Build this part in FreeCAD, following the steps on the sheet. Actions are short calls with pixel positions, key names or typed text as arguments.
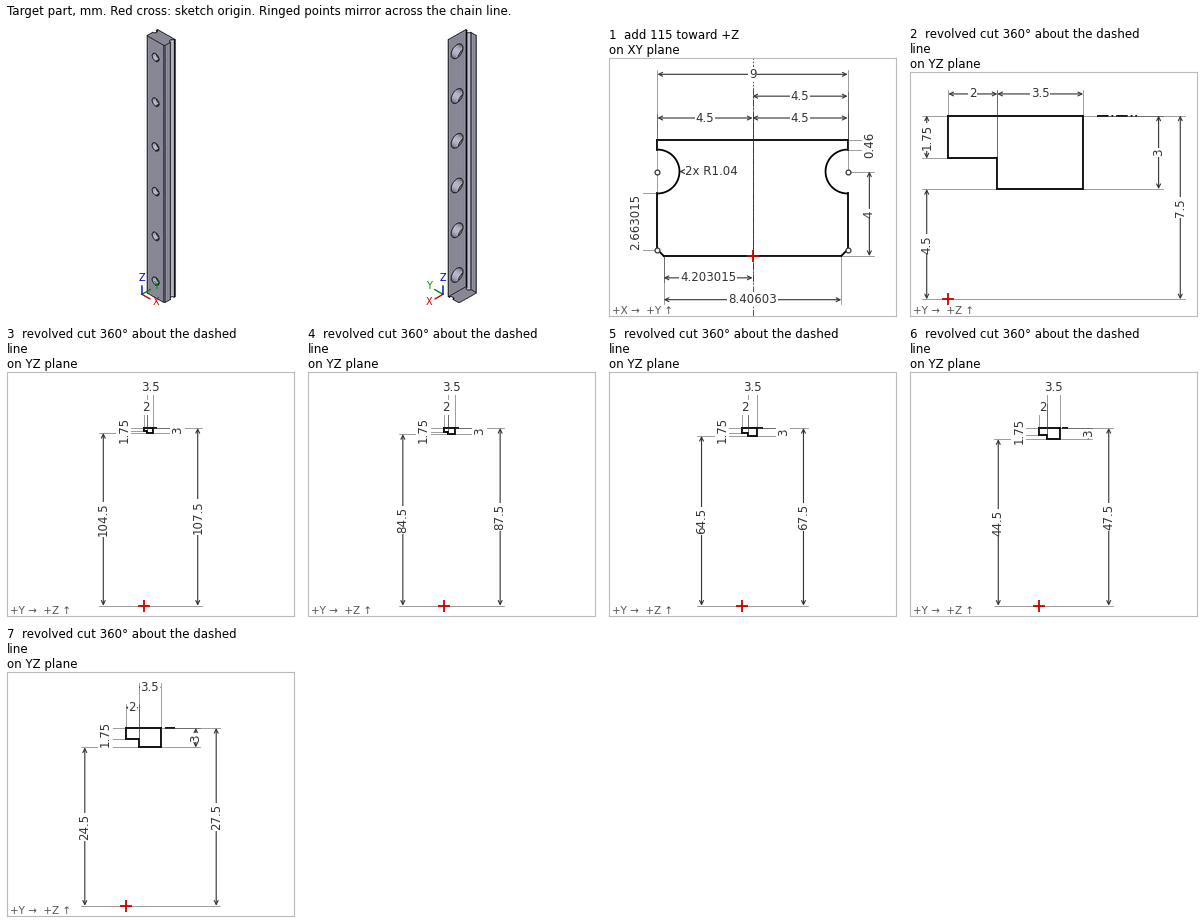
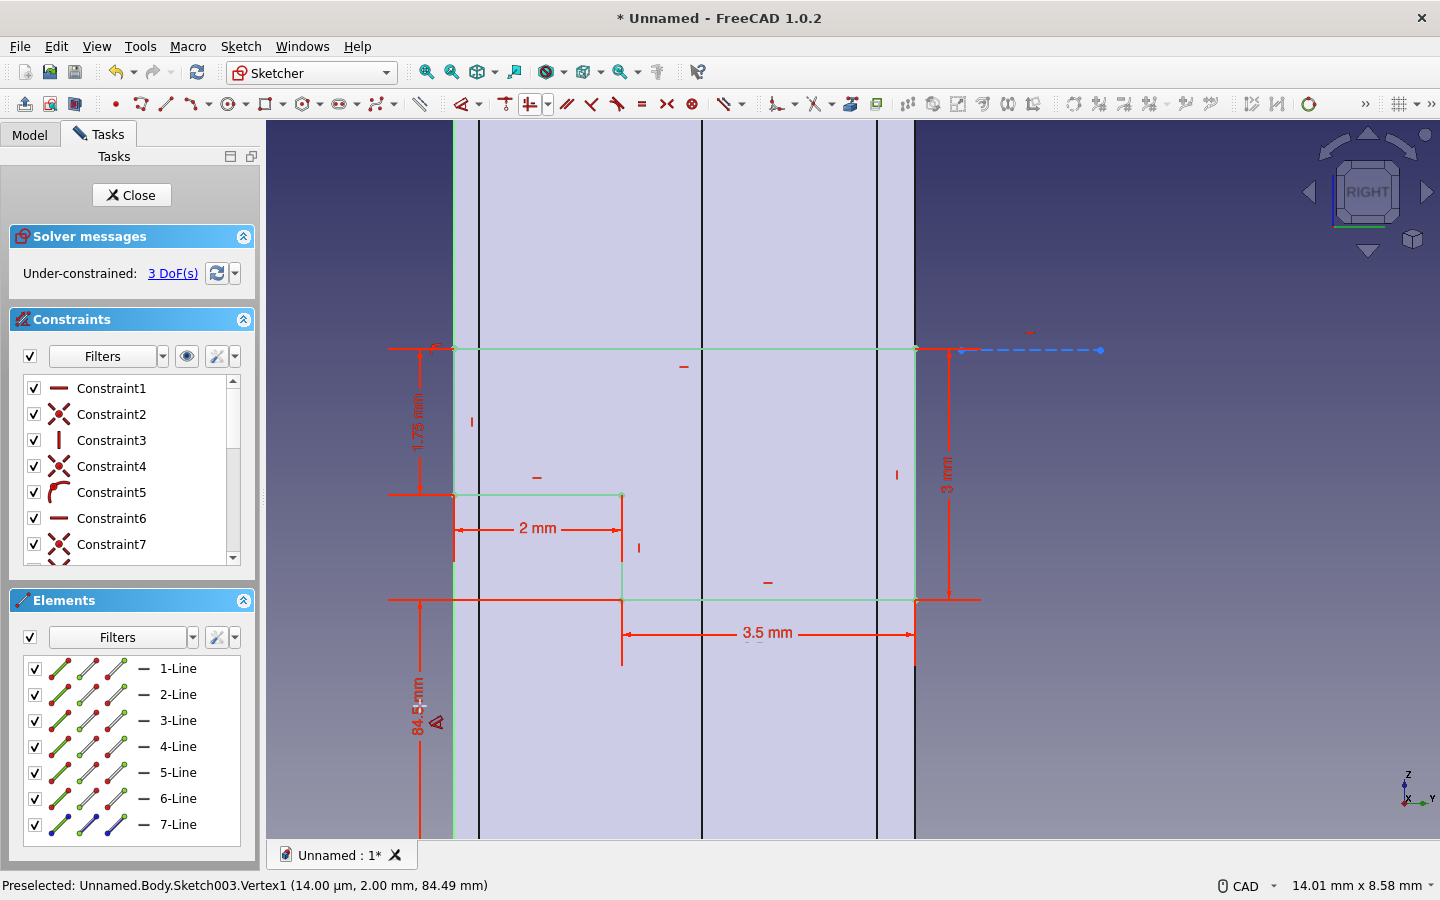
click(961, 350)
click(420, 581)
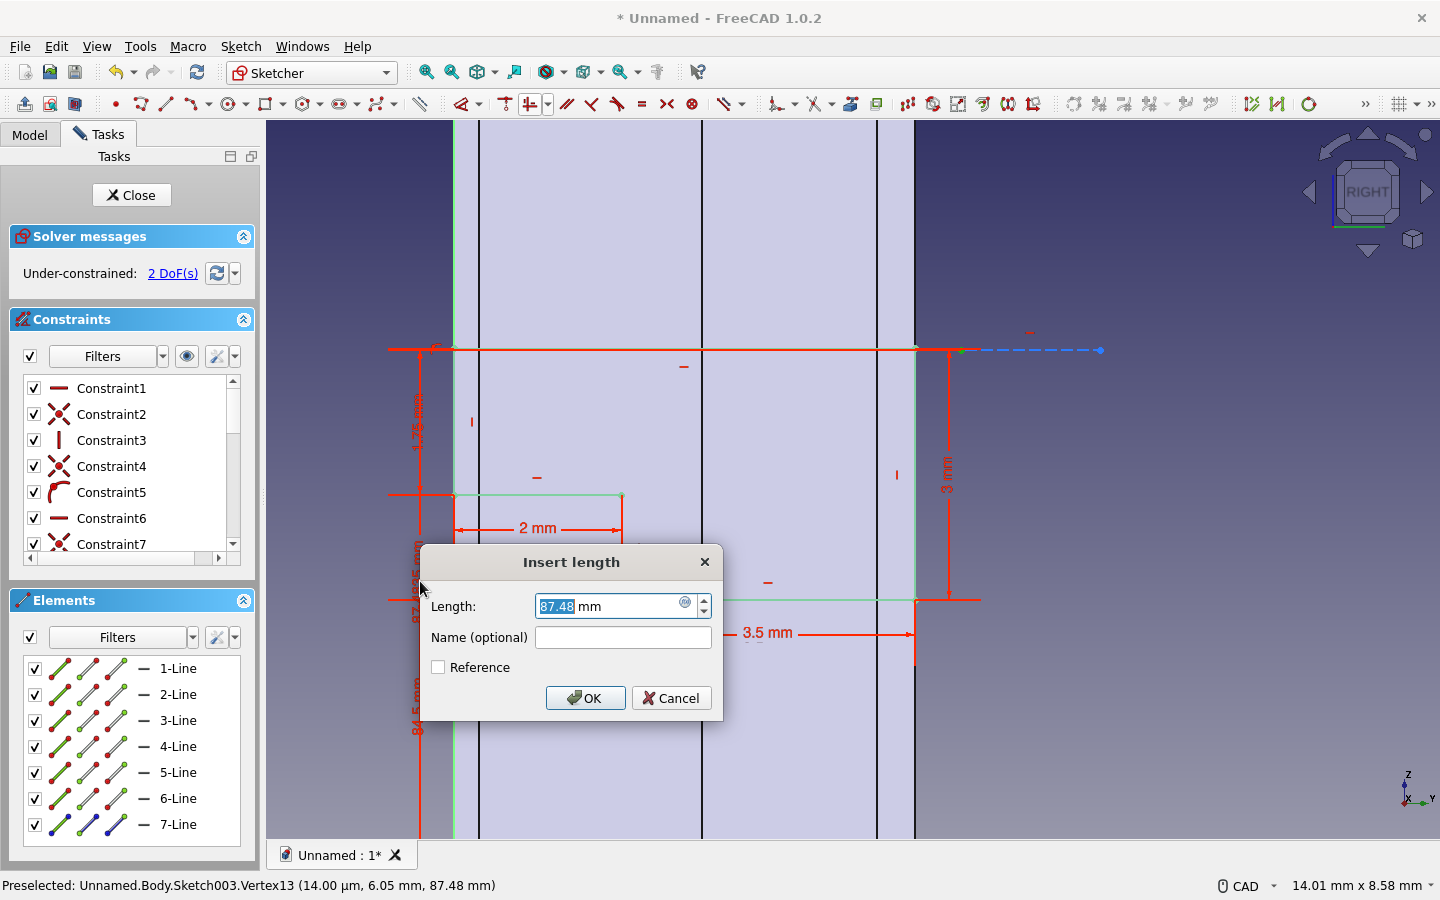
text(87.5)
key(Return)
key(Escape)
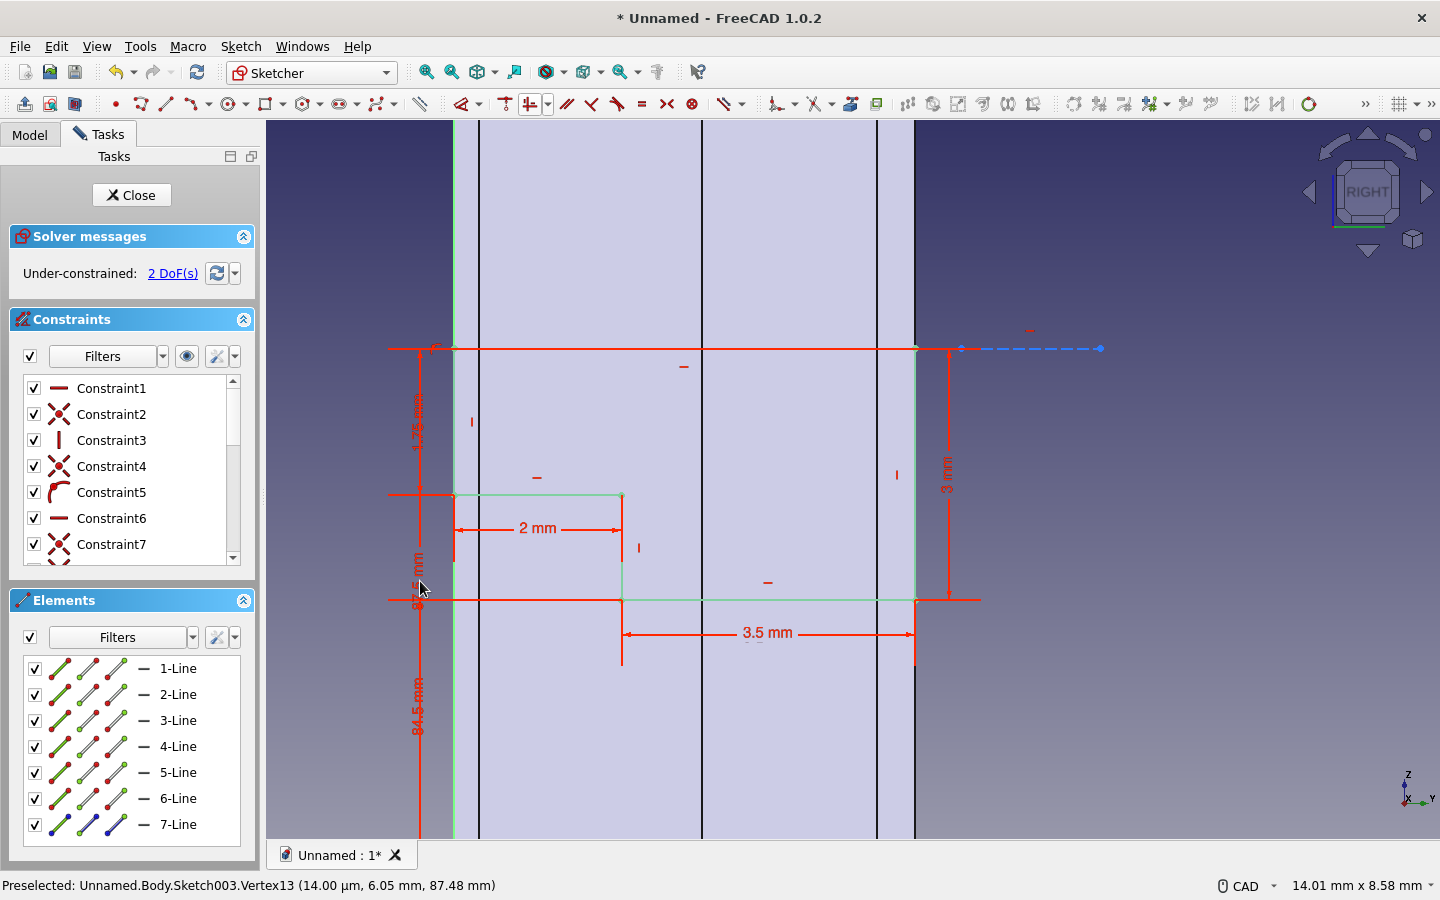
click(132, 195)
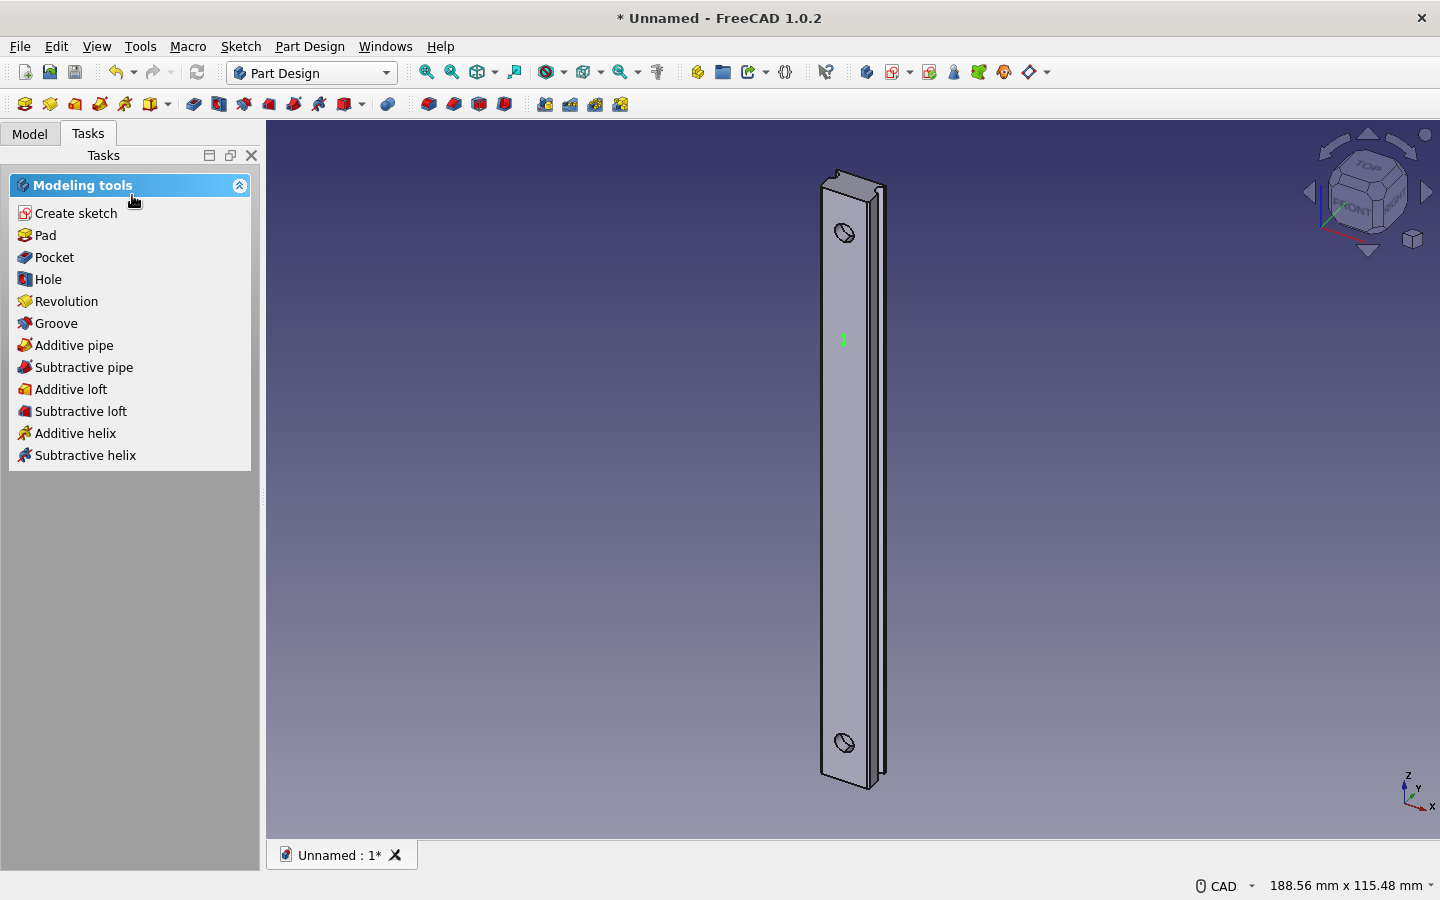
click(244, 104)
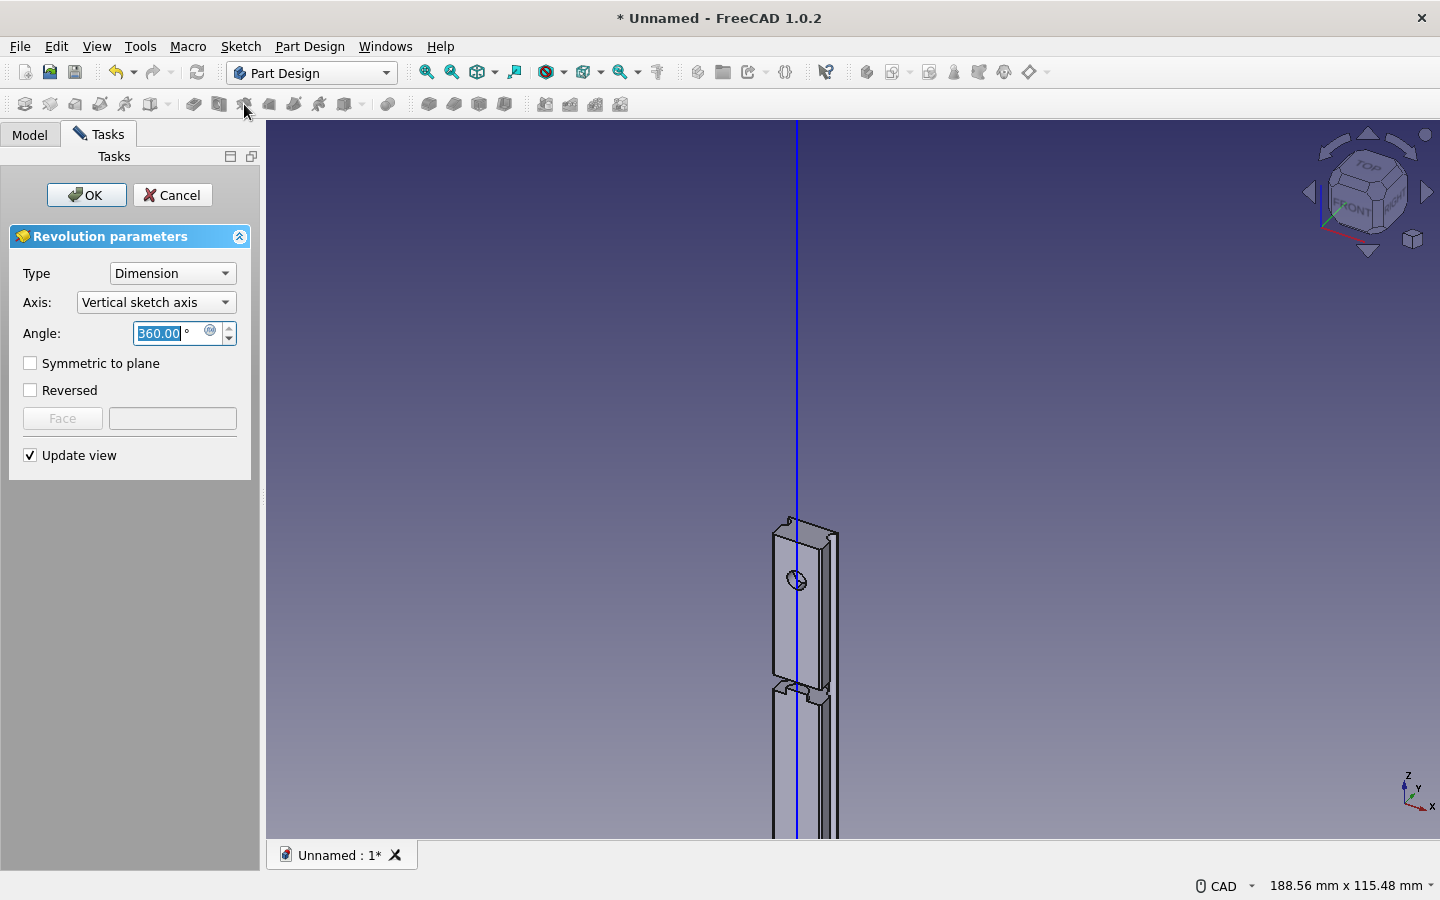
click(157, 302)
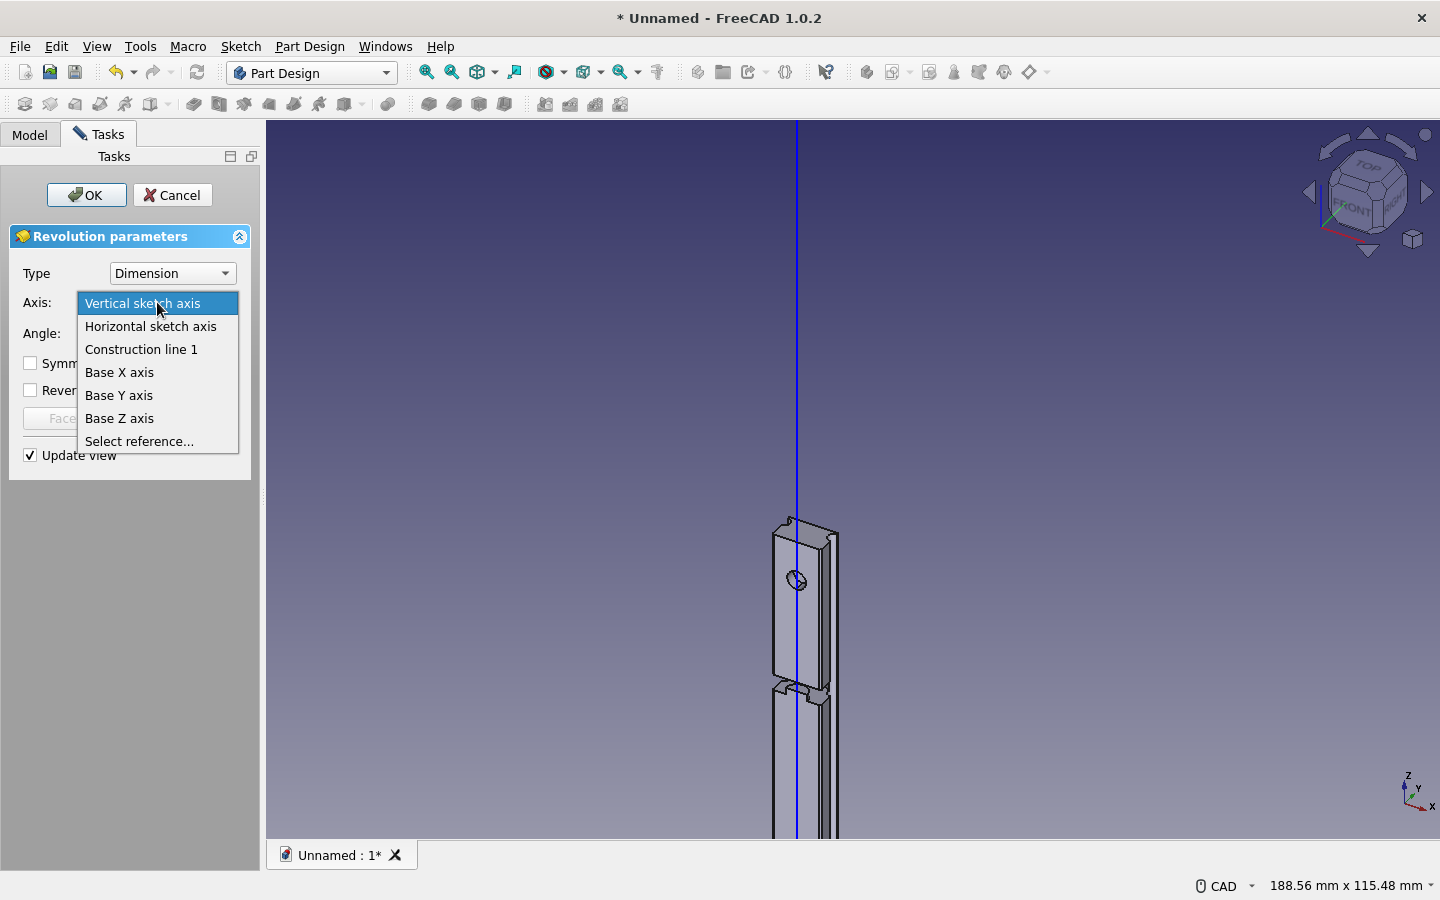
click(156, 350)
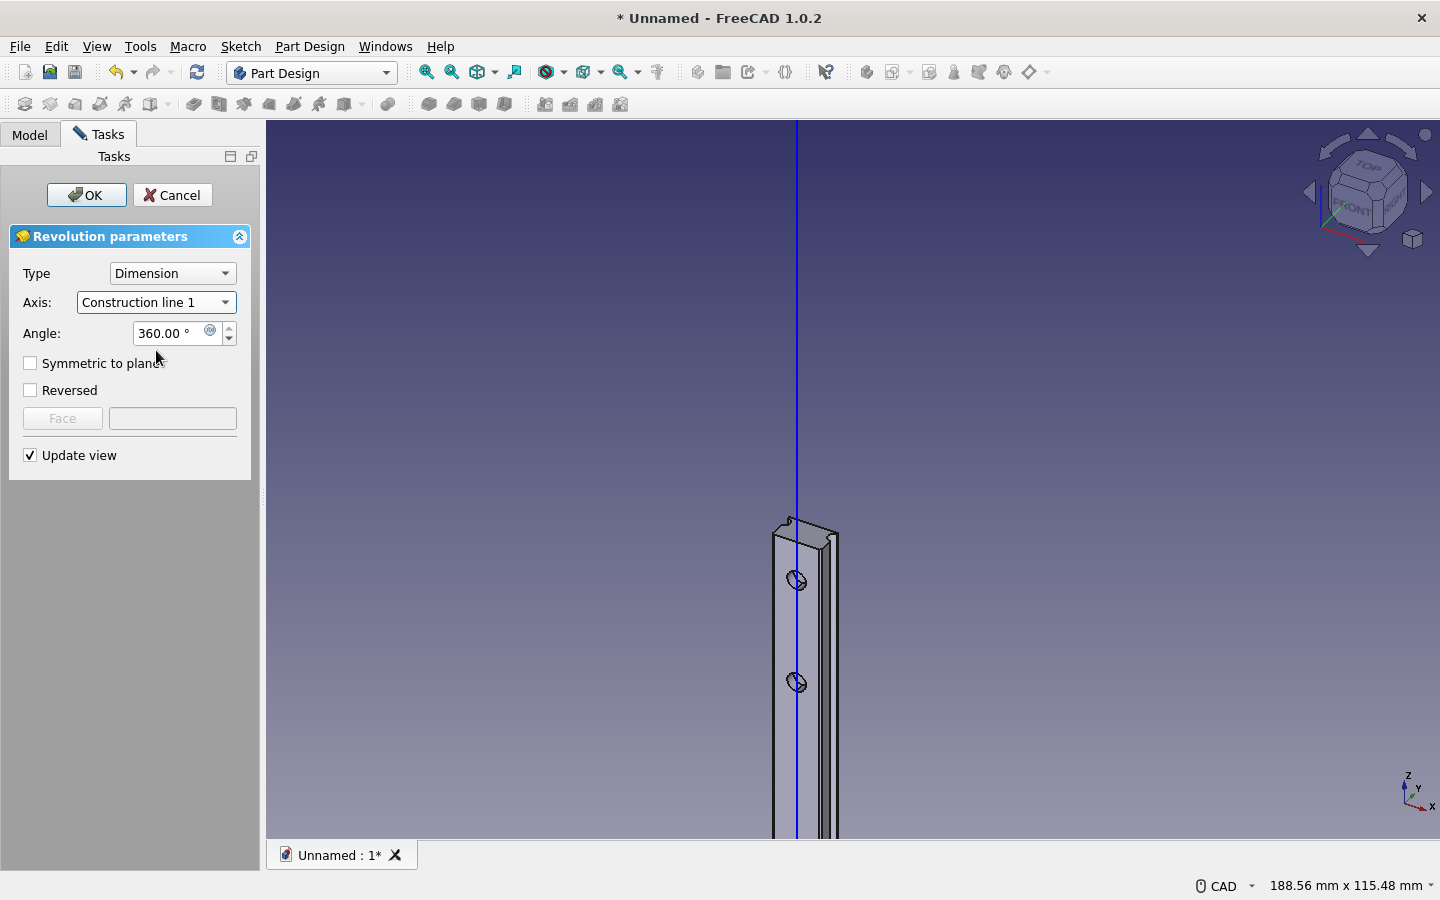
click(87, 195)